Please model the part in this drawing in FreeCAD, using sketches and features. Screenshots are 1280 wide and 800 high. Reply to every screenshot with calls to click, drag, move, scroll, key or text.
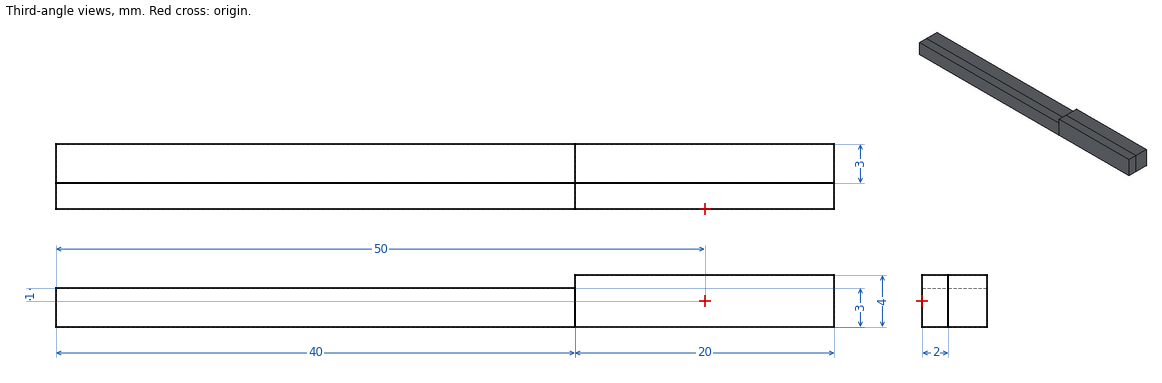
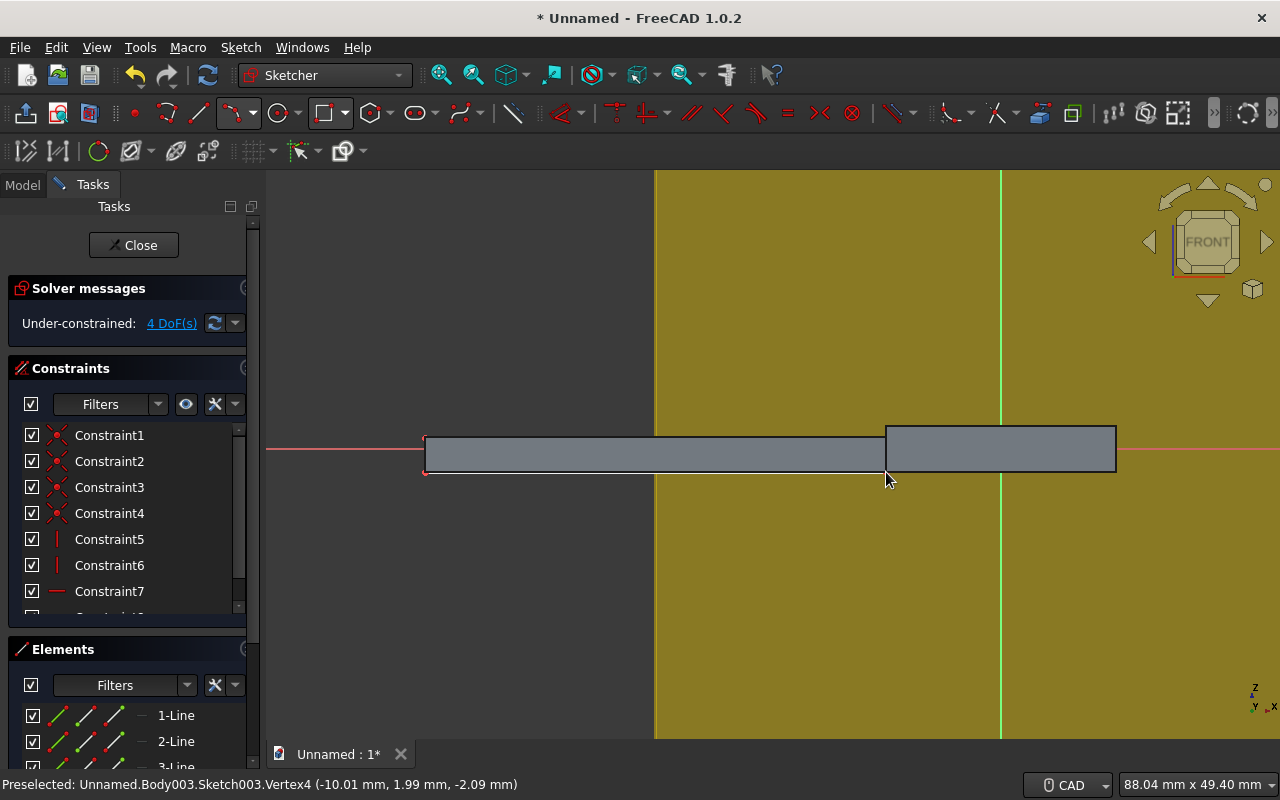
click(560, 114)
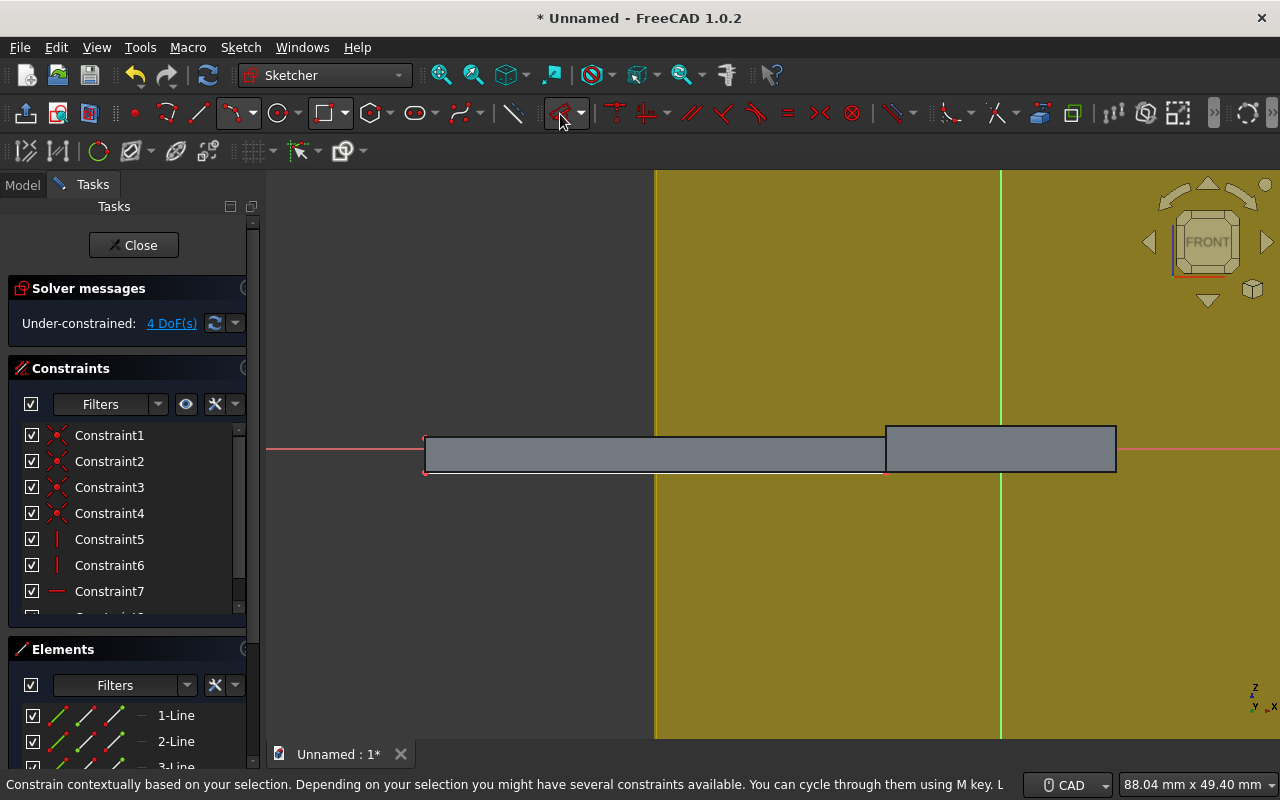
scroll(425, 449, up, 2)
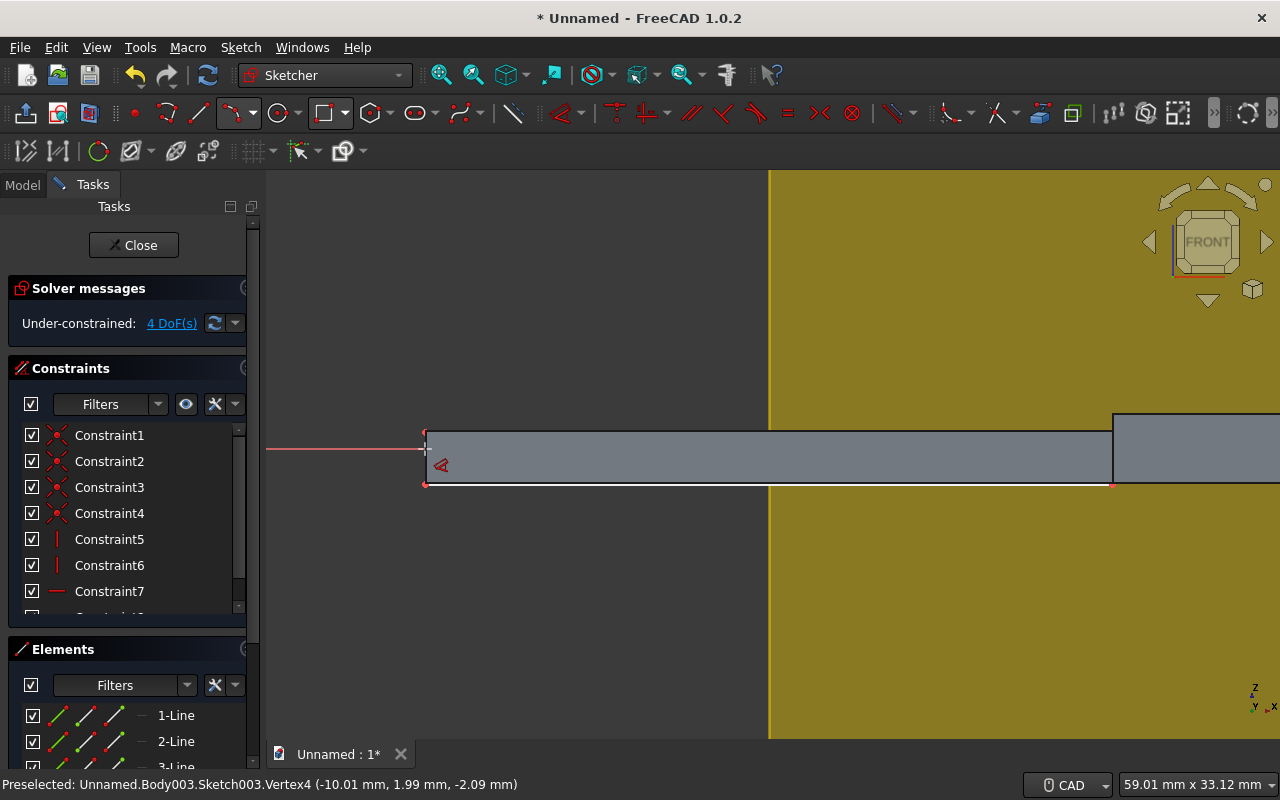
click(426, 448)
click(392, 471)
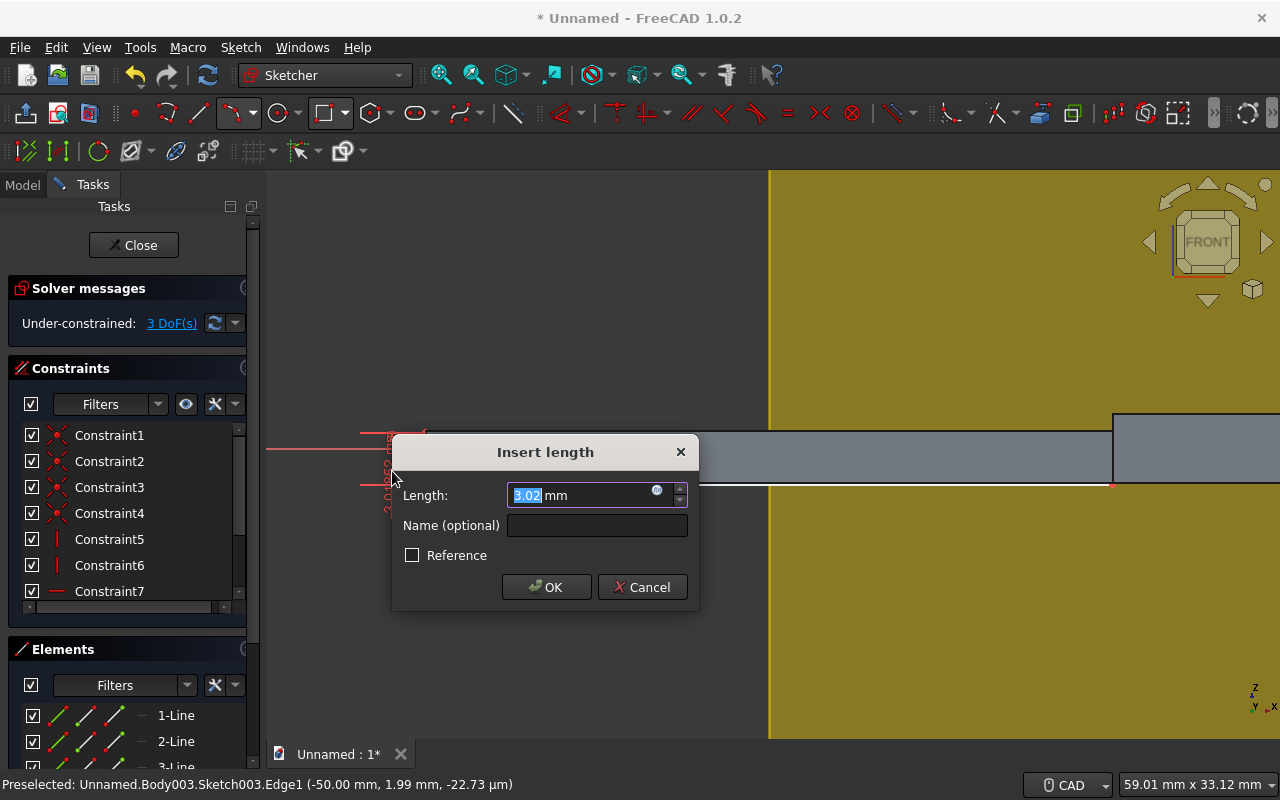
text(3)
key(Return)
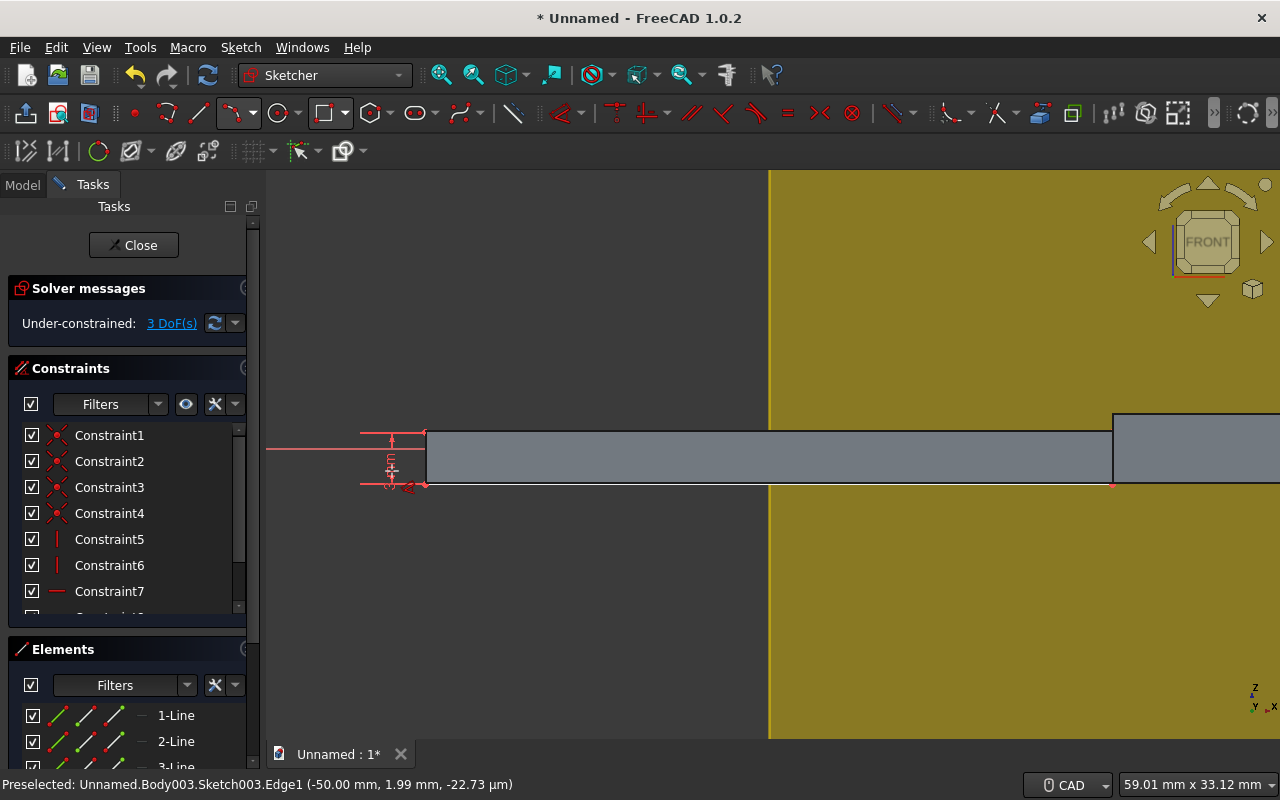
click(632, 484)
click(769, 518)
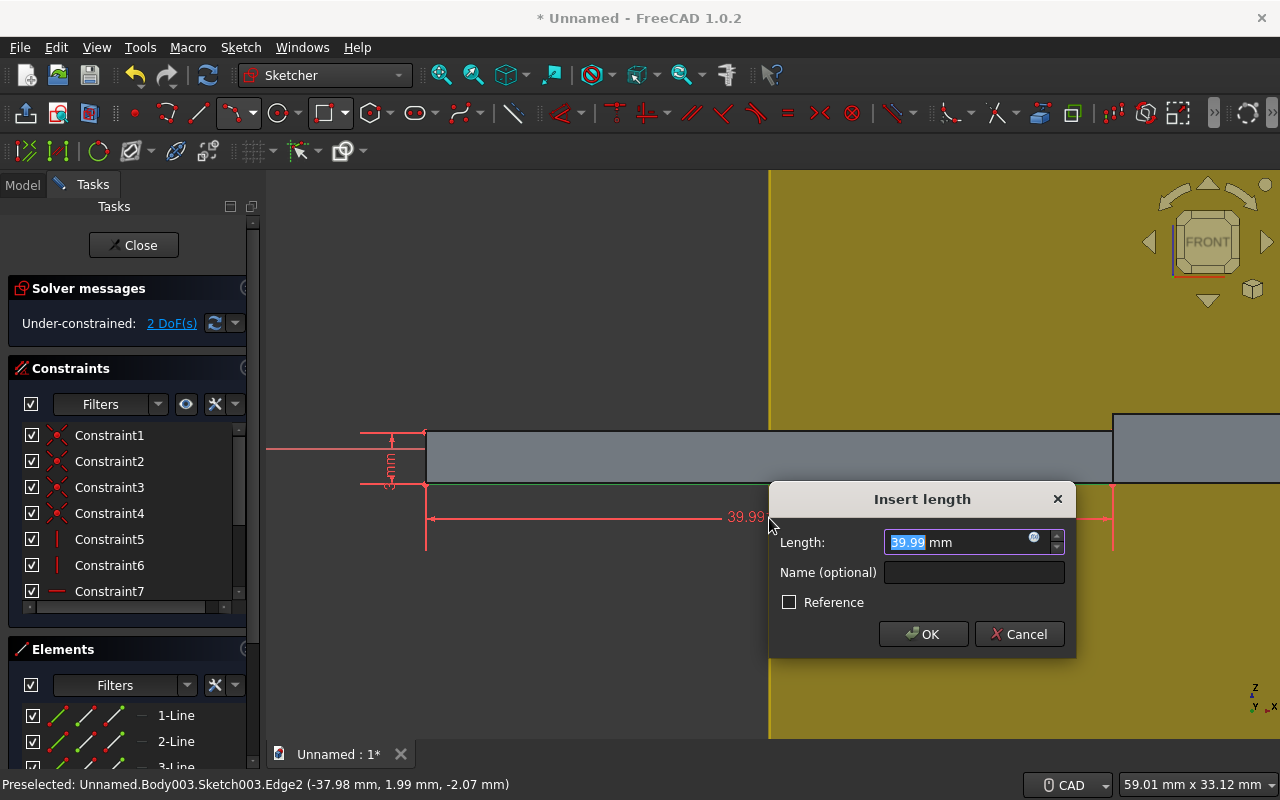
text(40)
key(Return)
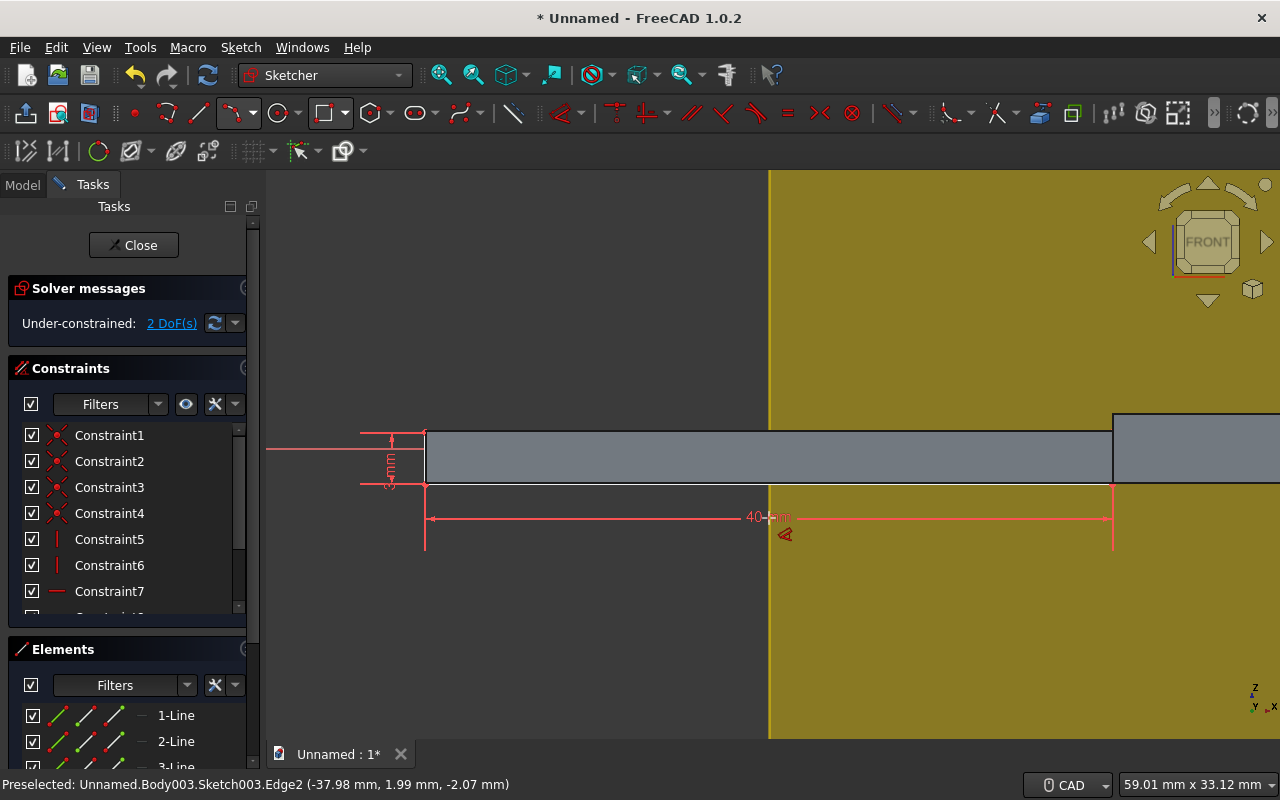
scroll(425, 433, up, 5)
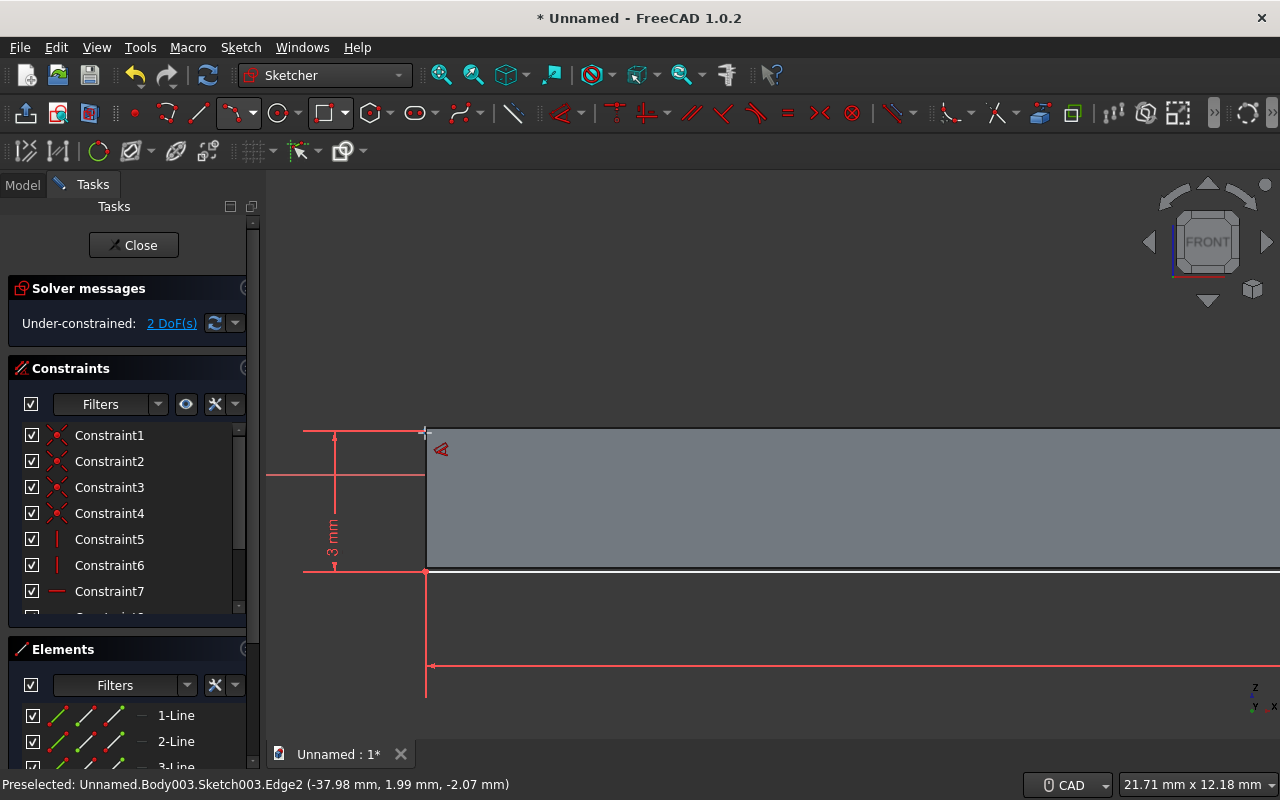
click(426, 431)
click(392, 453)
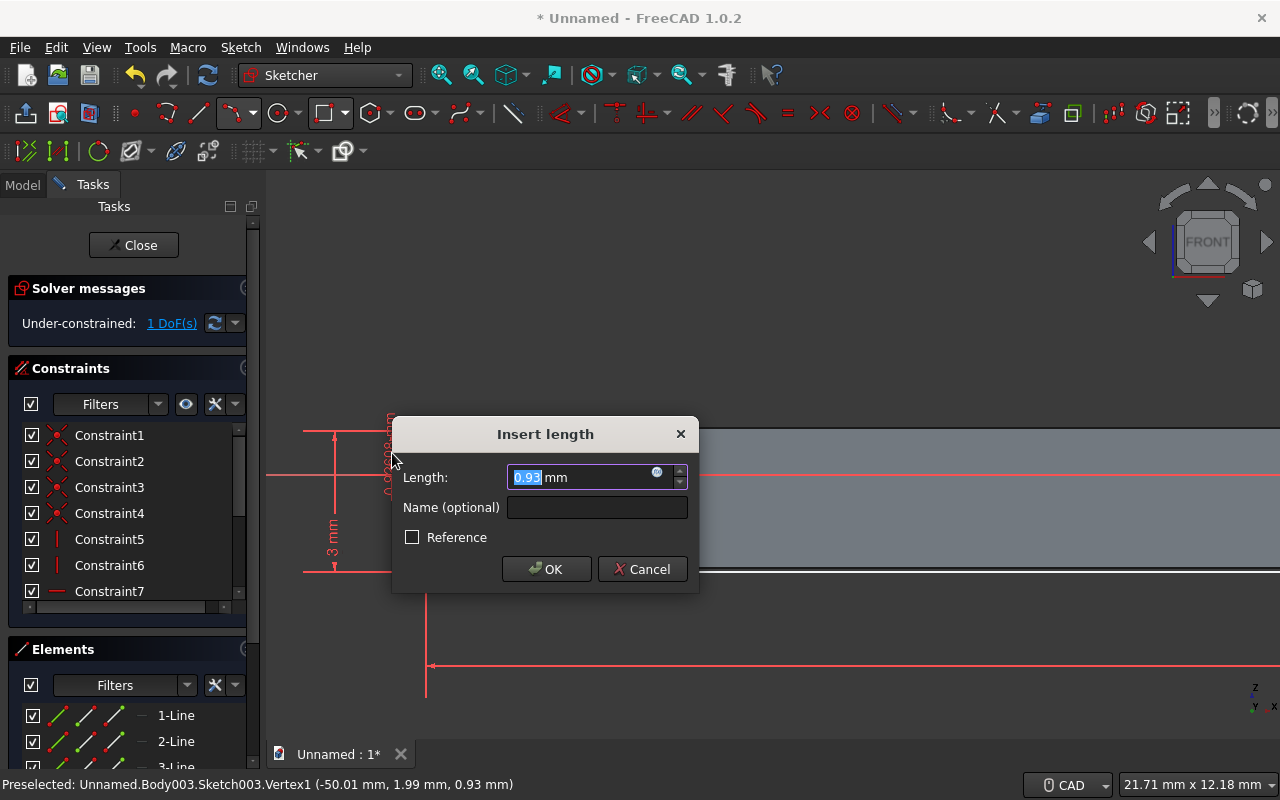
text(1)
key(Return)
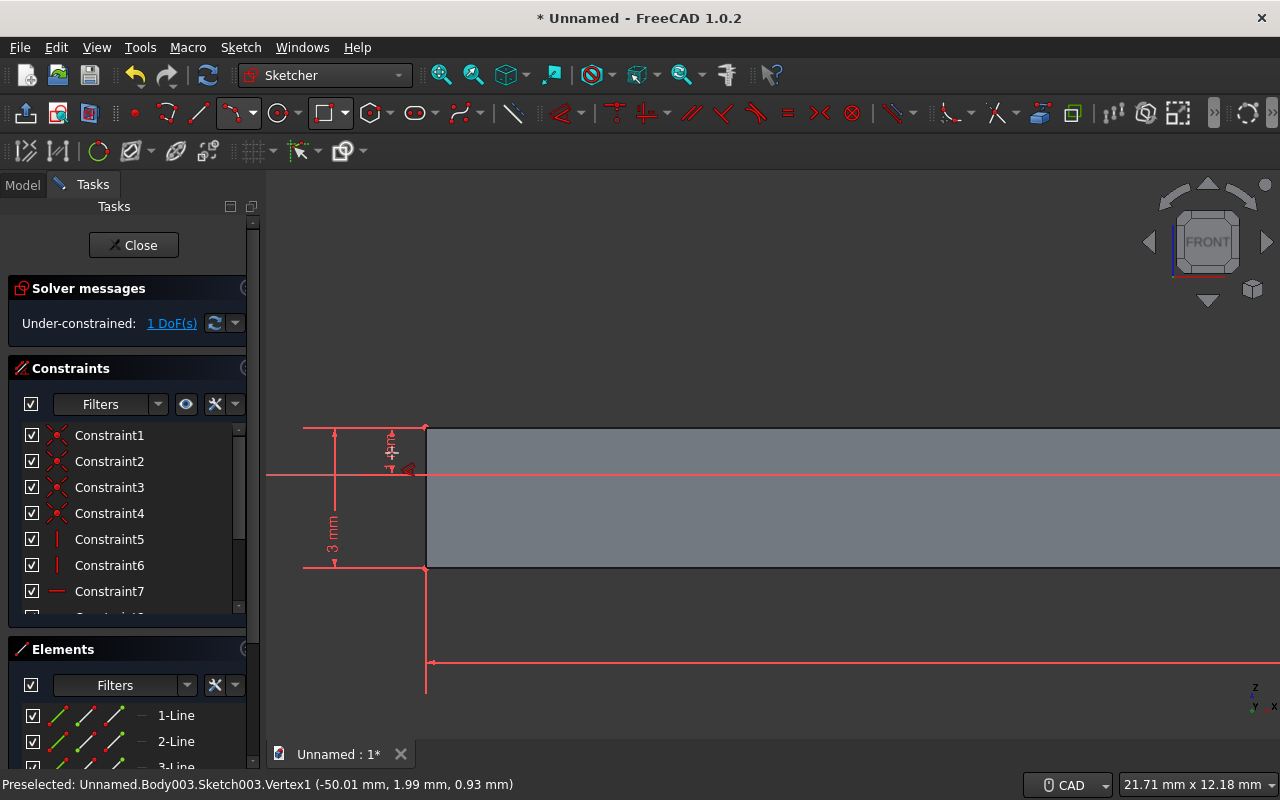
scroll(413, 440, down, 7)